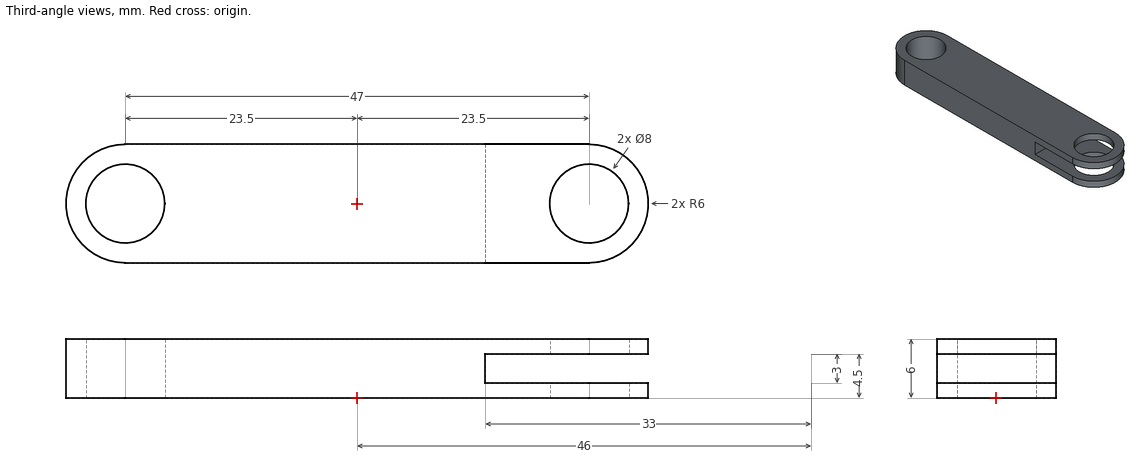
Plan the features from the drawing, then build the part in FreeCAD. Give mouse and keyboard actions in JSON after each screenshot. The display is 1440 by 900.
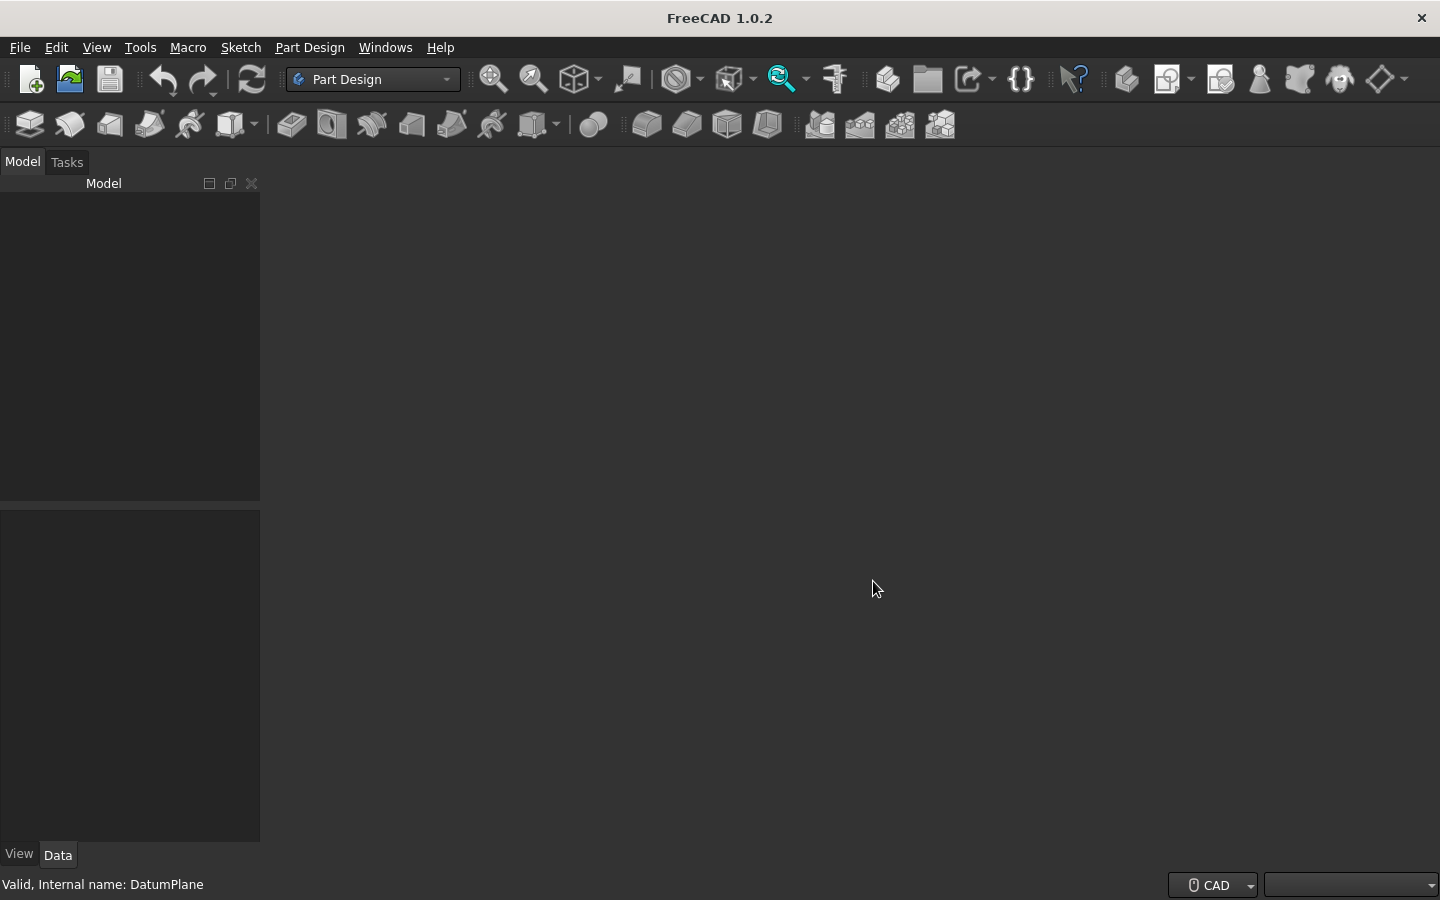
{"action": "key", "text": "ctrl+n"}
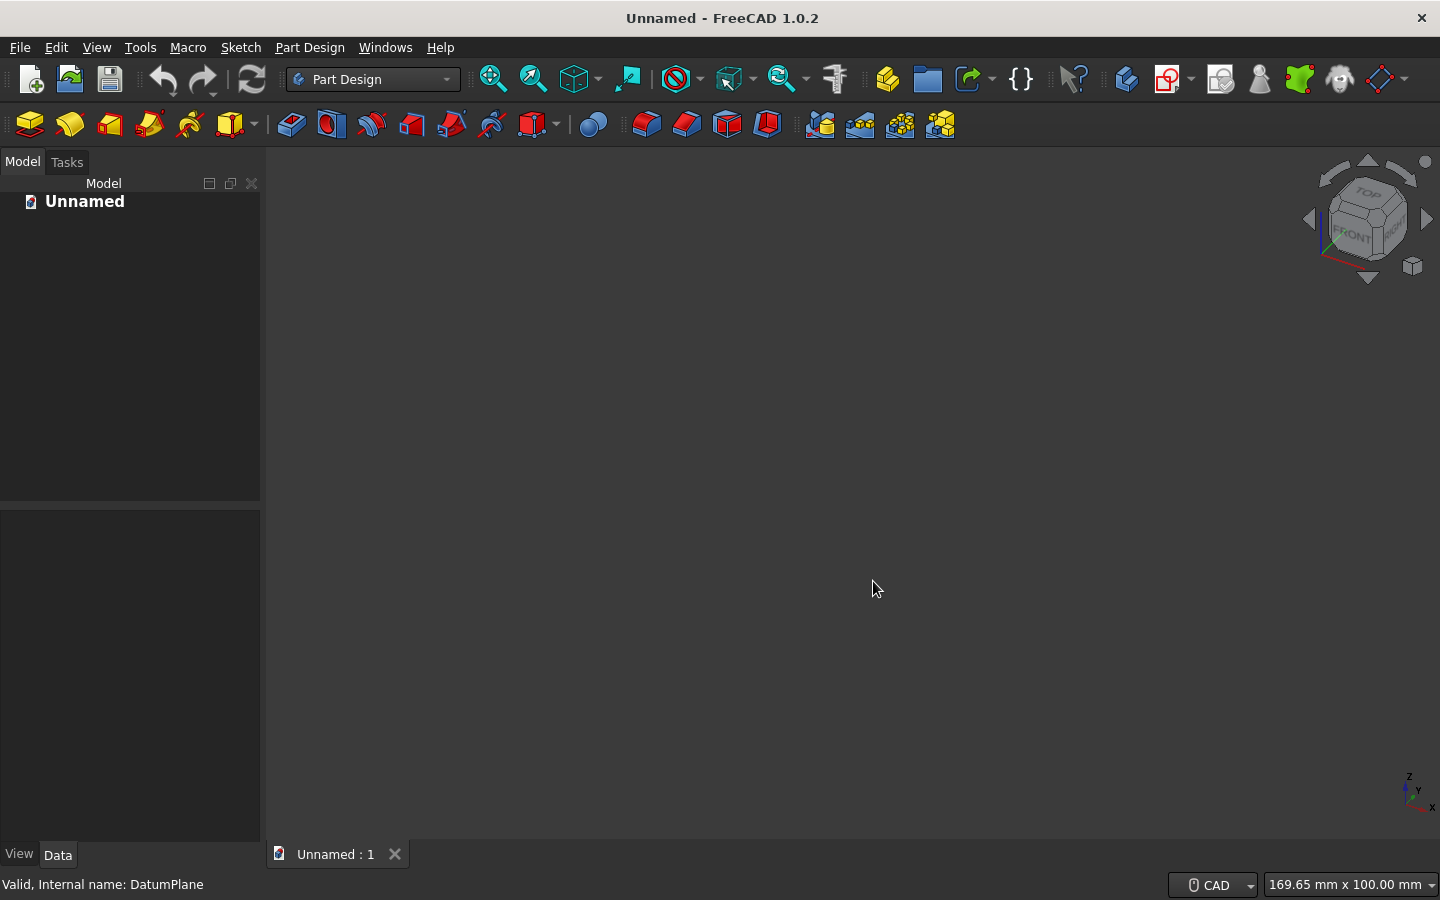
{"action": "left_click", "coordinate": [1168, 80]}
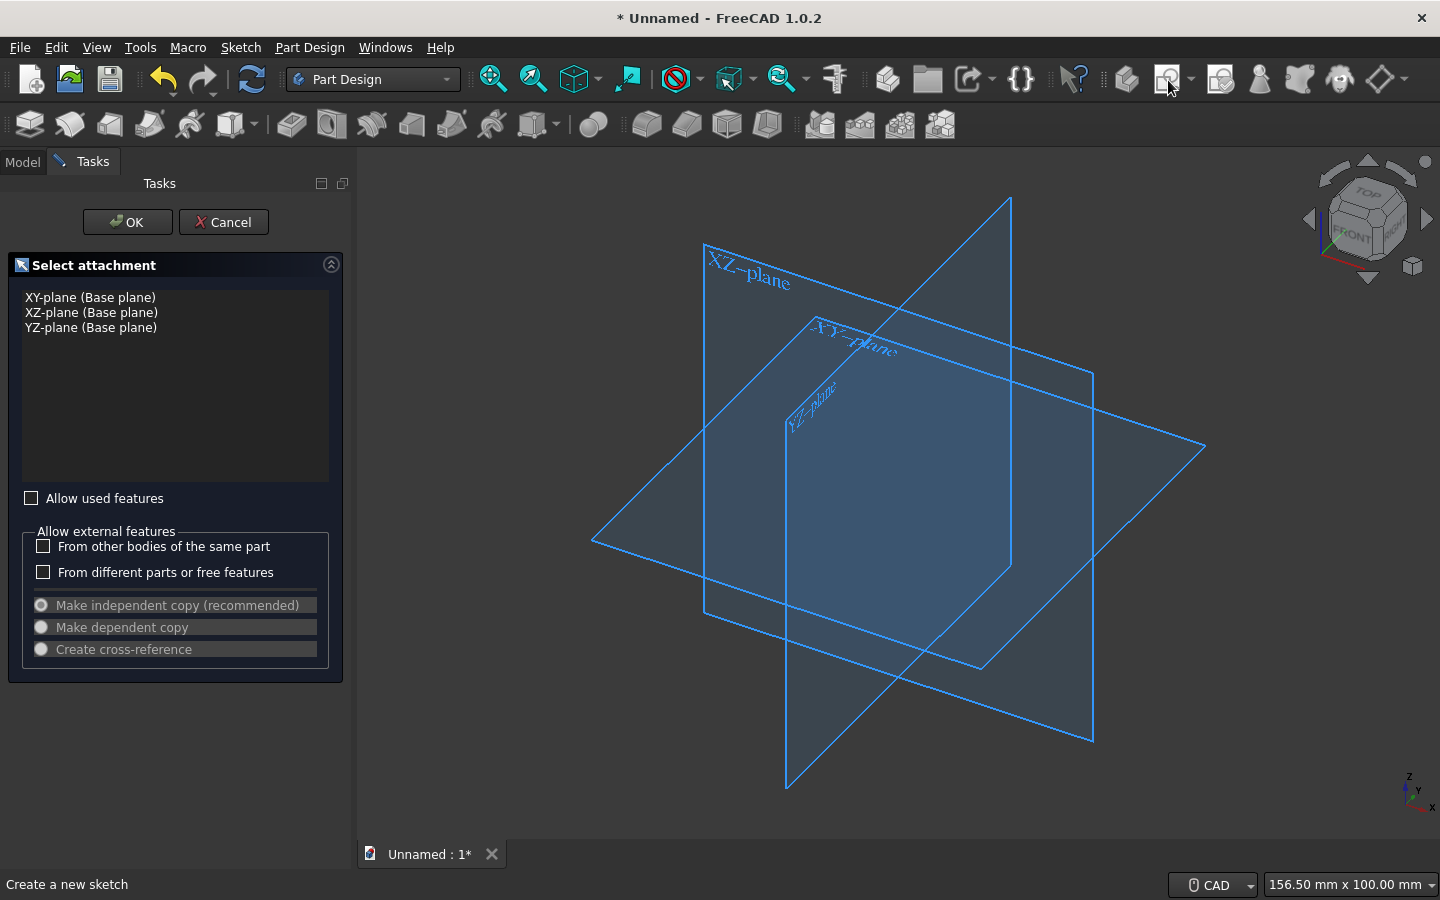
{"action": "left_click", "coordinate": [82, 298]}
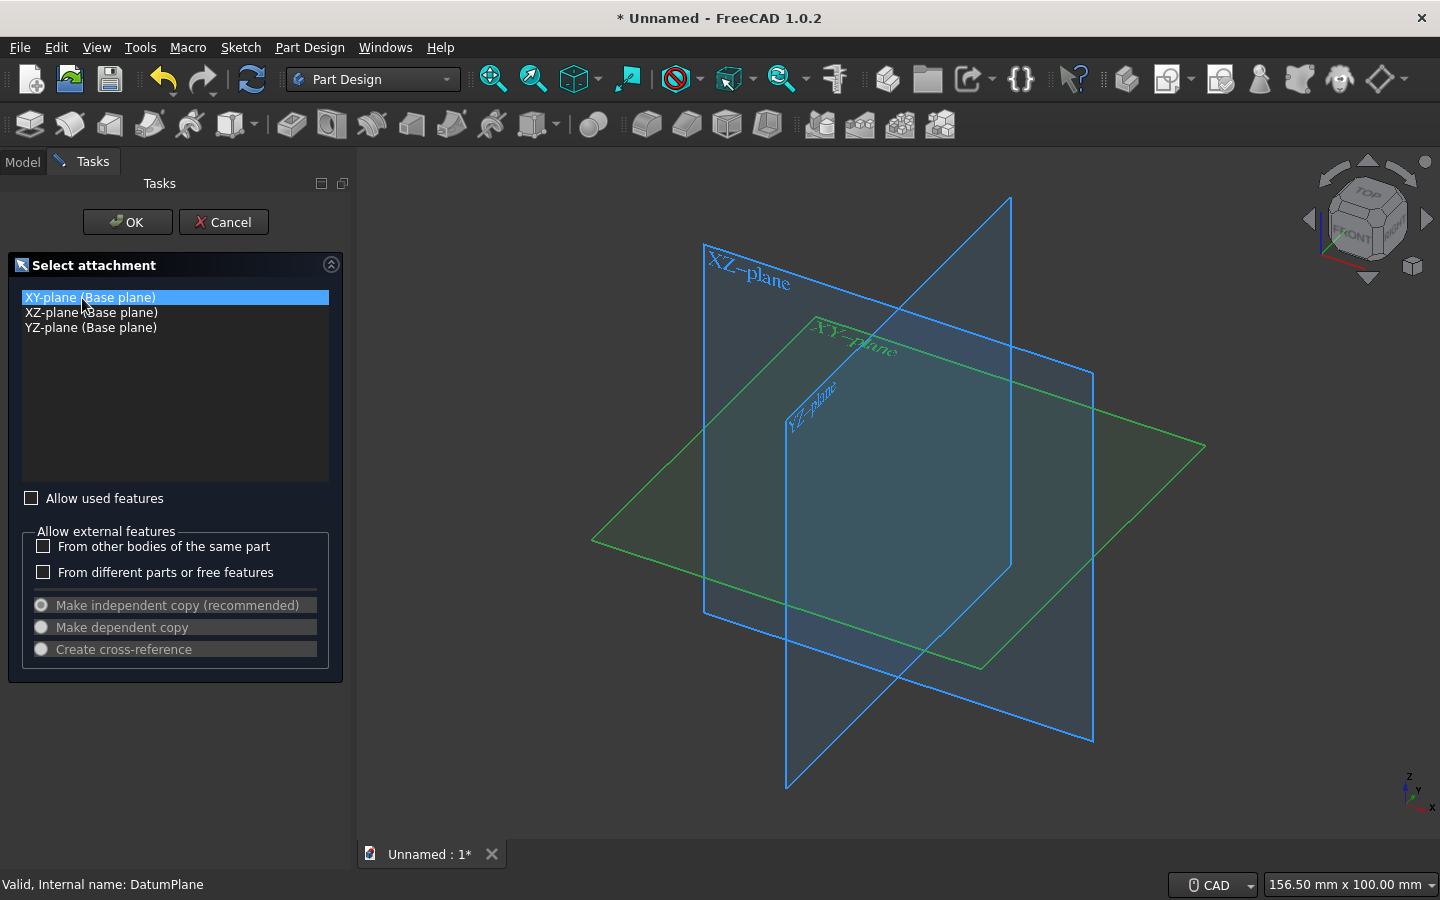
{"action": "left_click", "coordinate": [128, 222]}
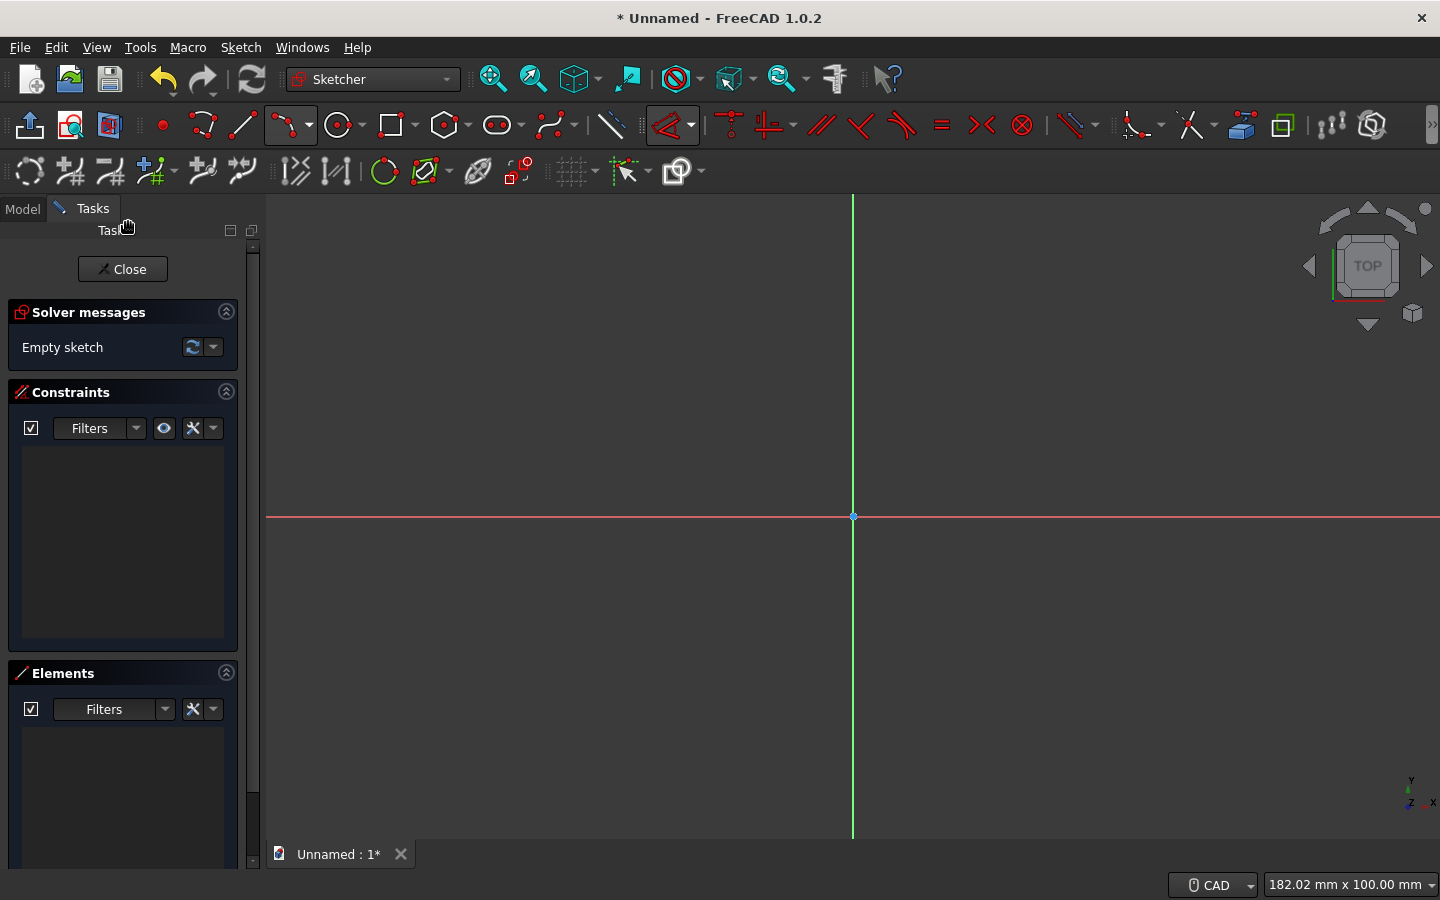
{"action": "scroll", "coordinate": [936, 516], "scroll_direction": "up", "scroll_amount": 3}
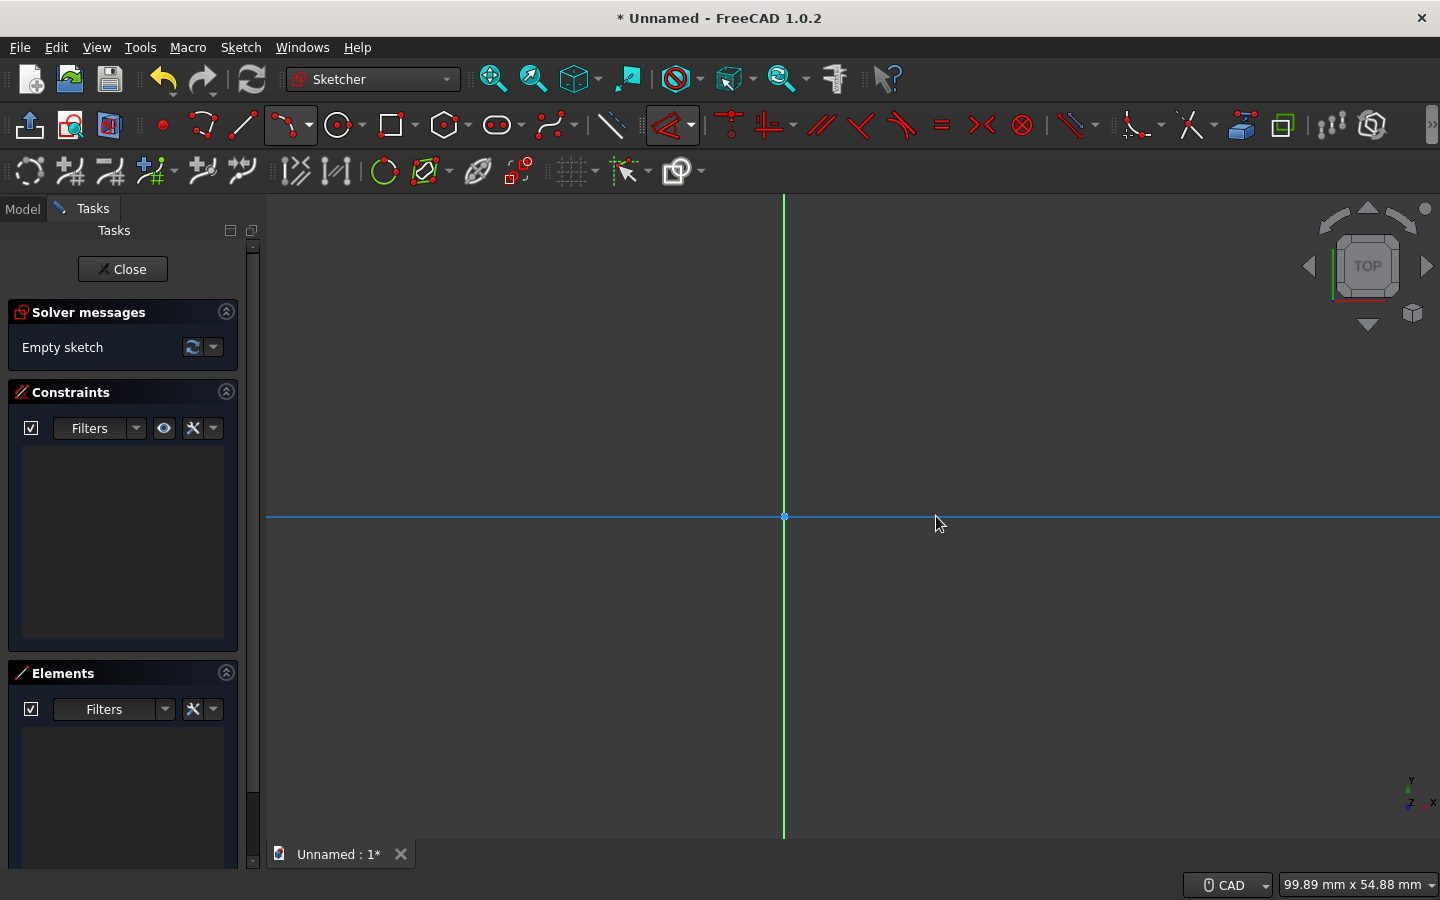
{"action": "left_click", "coordinate": [498, 126]}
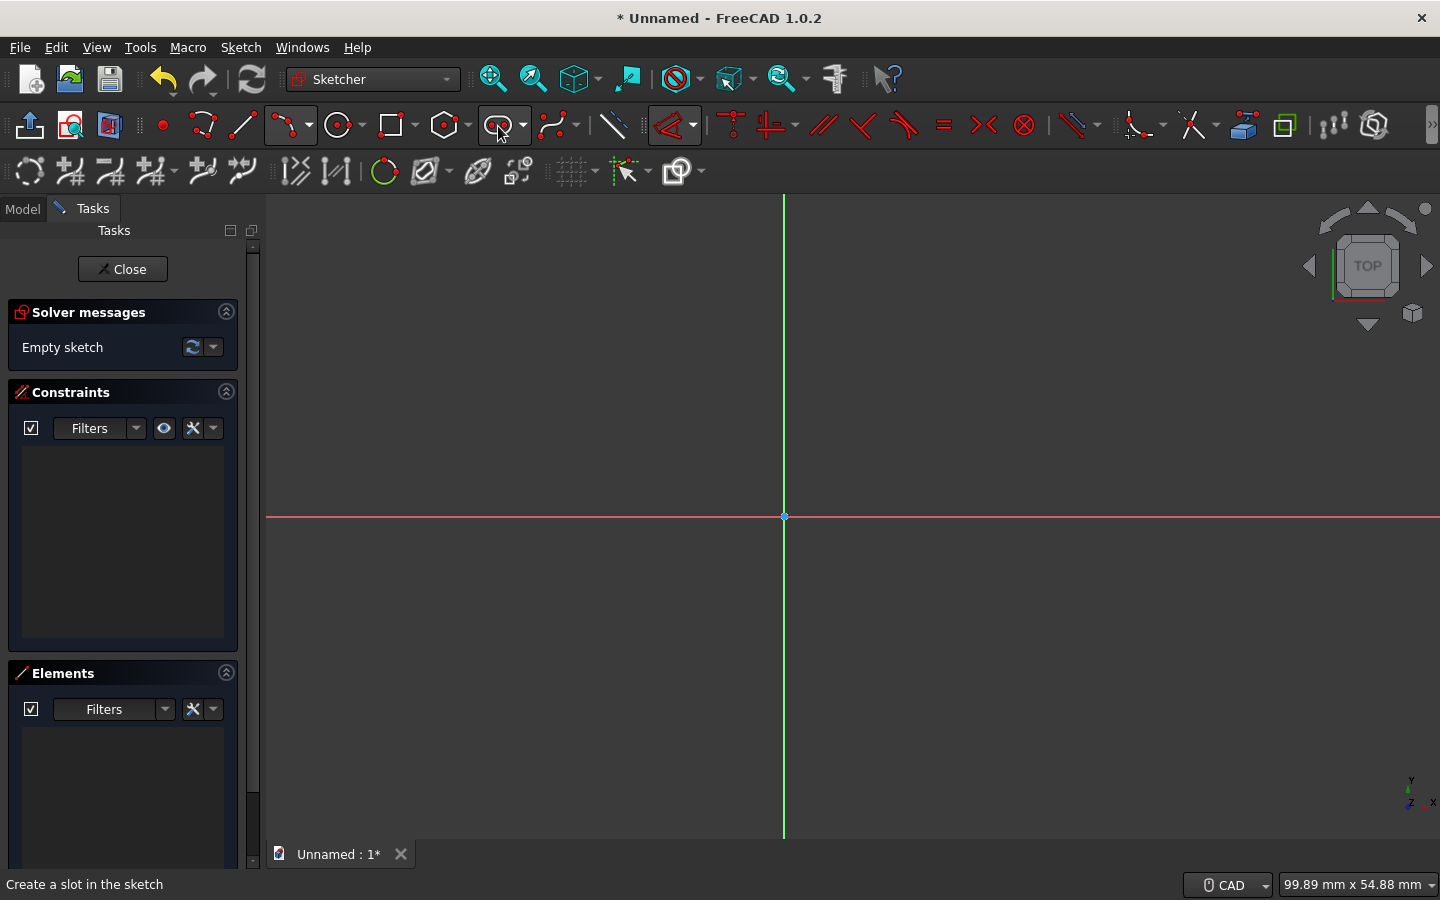
{"action": "left_click", "coordinate": [508, 516]}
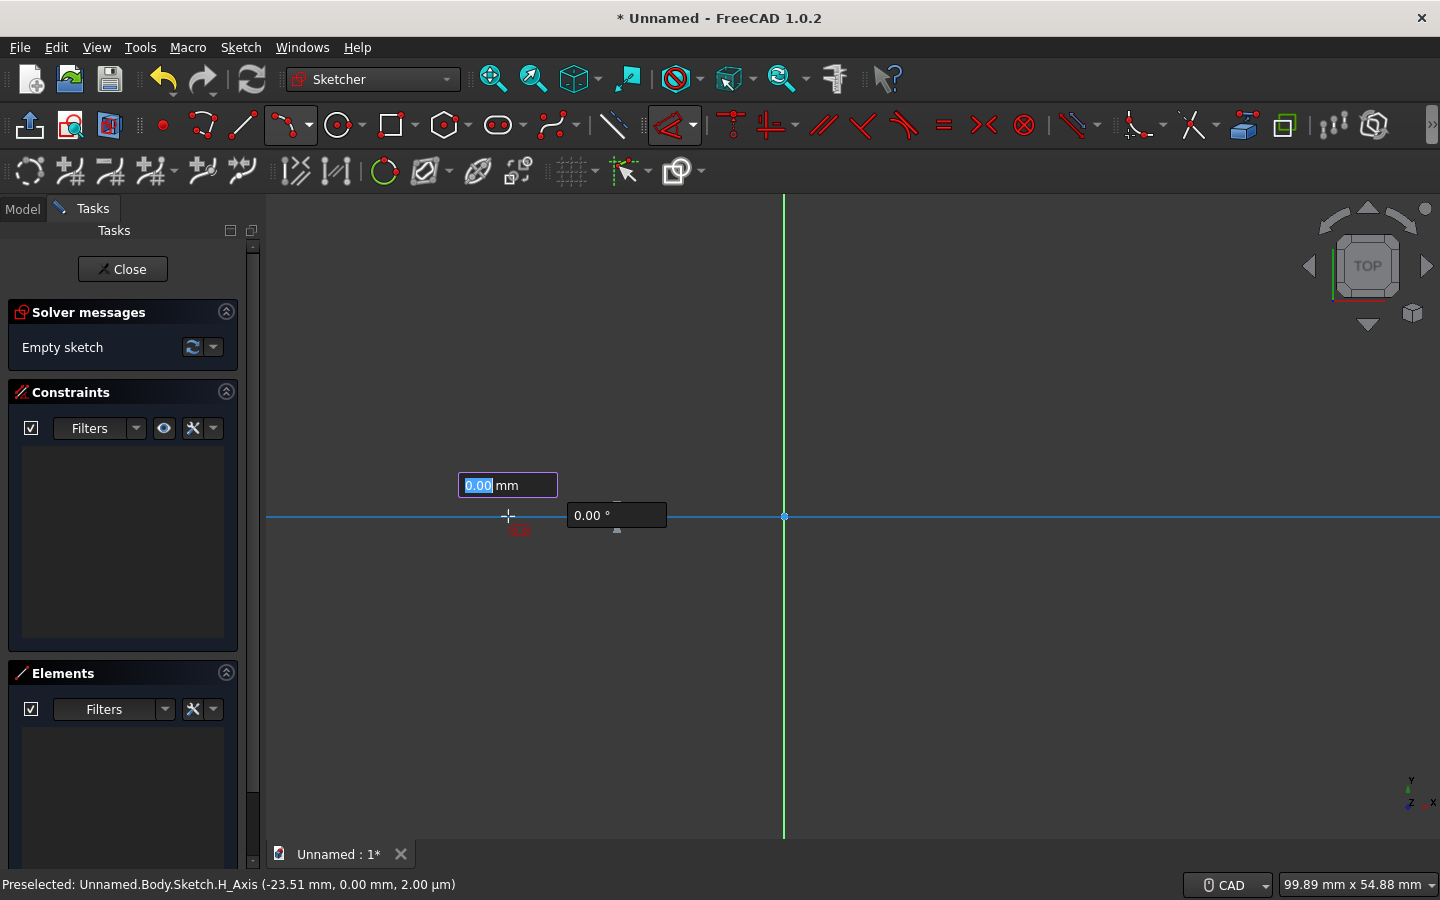
{"action": "left_click", "coordinate": [1060, 508]}